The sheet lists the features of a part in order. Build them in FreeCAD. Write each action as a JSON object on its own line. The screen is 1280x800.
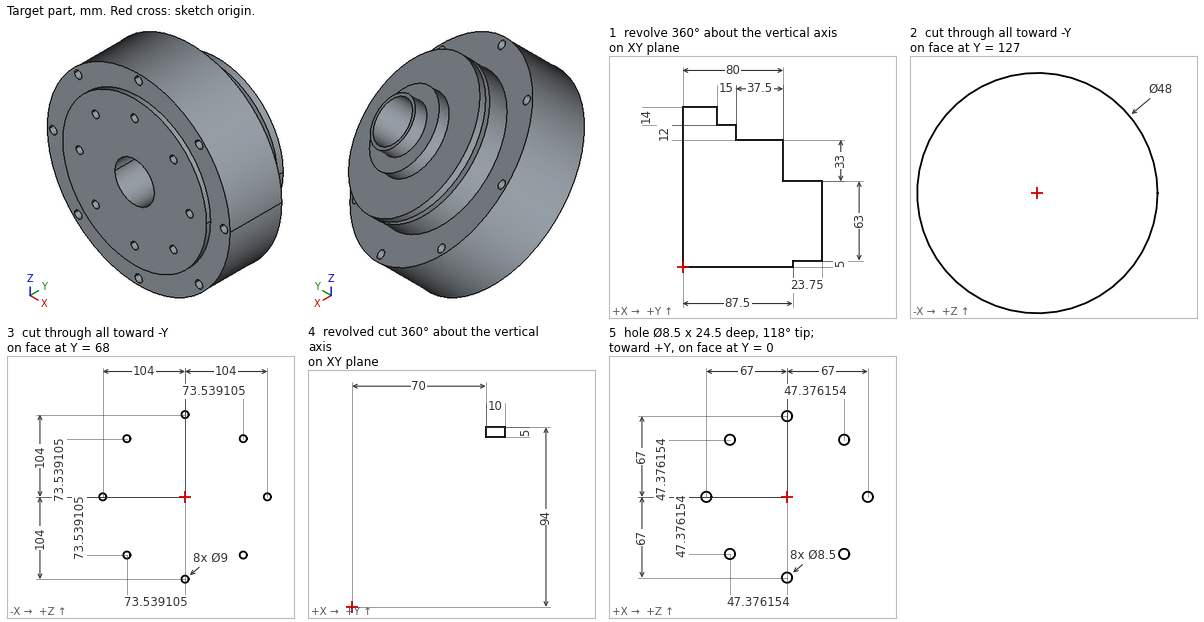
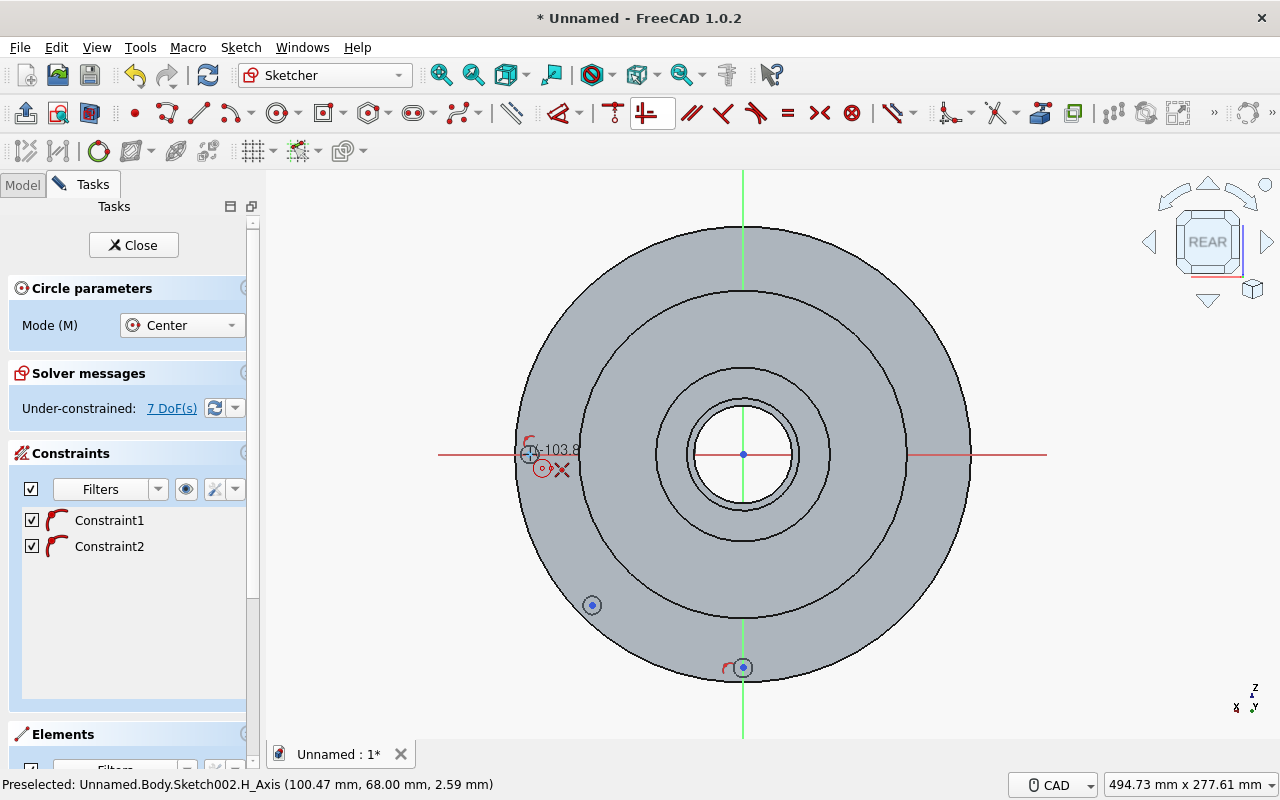
{"action": "scroll", "coordinate": [581, 331], "scroll_direction": "up", "scroll_amount": 6}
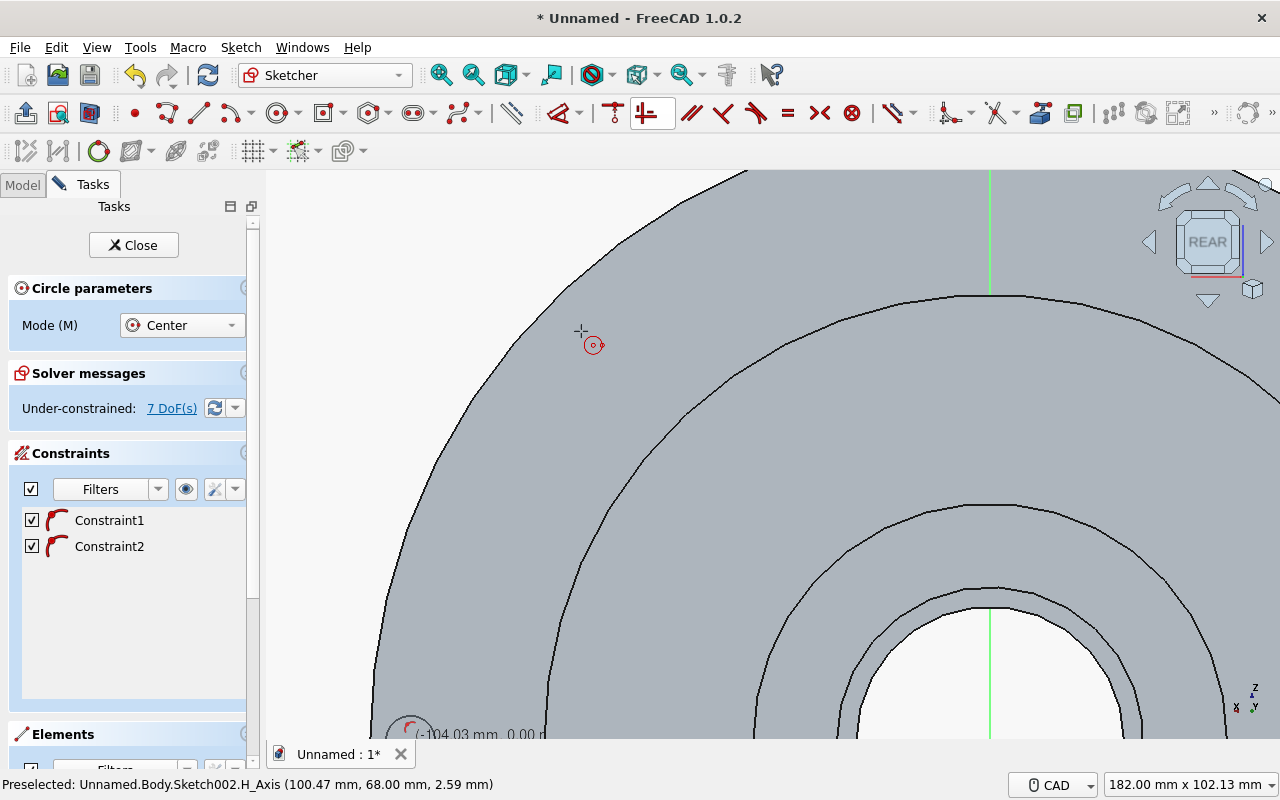
{"action": "left_click", "coordinate": [580, 331]}
{"action": "left_click", "coordinate": [598, 313]}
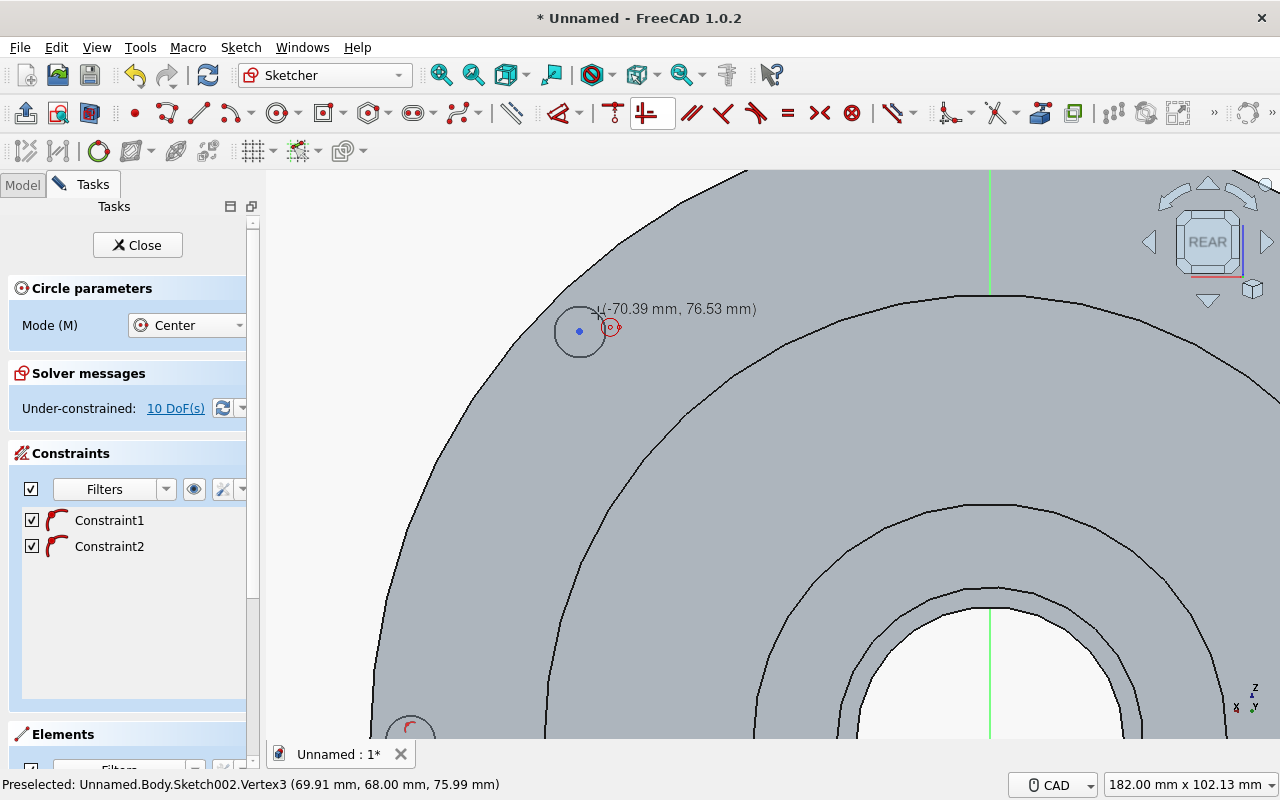
{"action": "scroll", "coordinate": [581, 331], "scroll_direction": "down", "scroll_amount": 6}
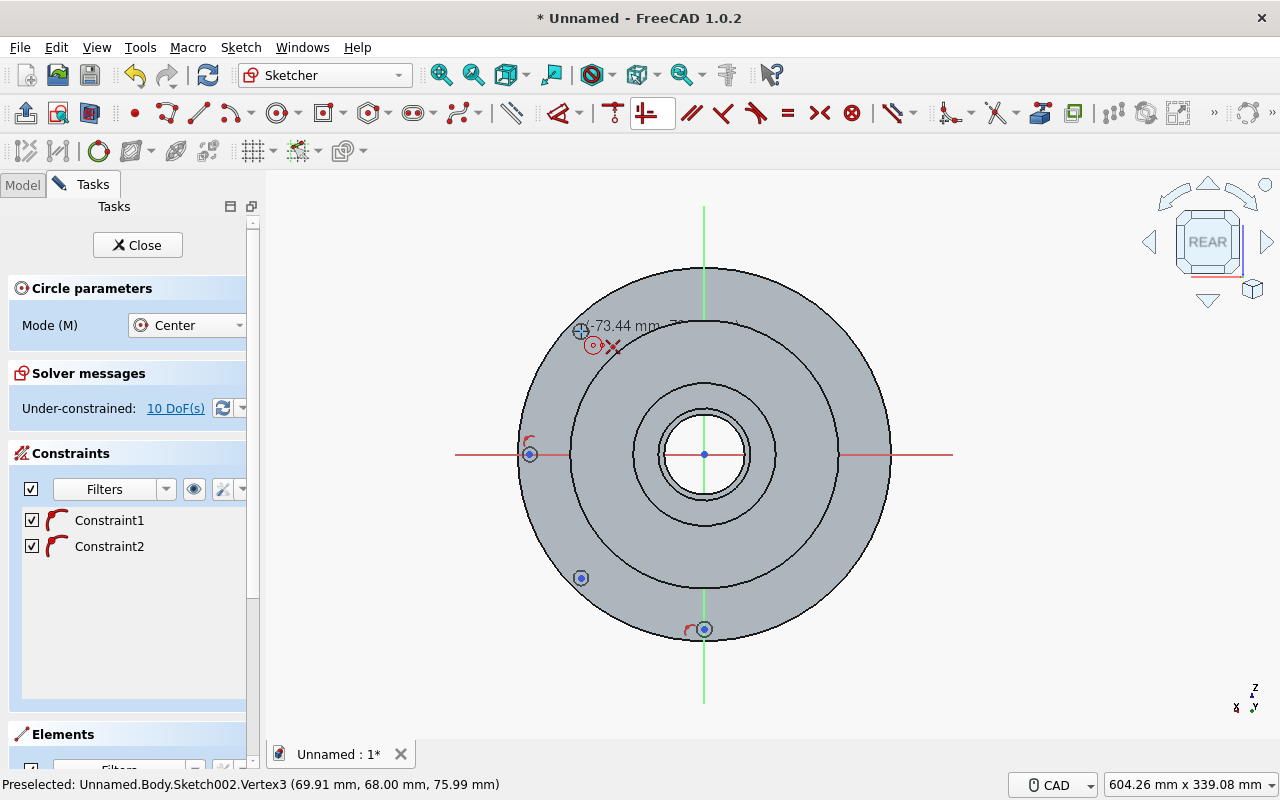
{"action": "scroll", "coordinate": [704, 280], "scroll_direction": "up", "scroll_amount": 6}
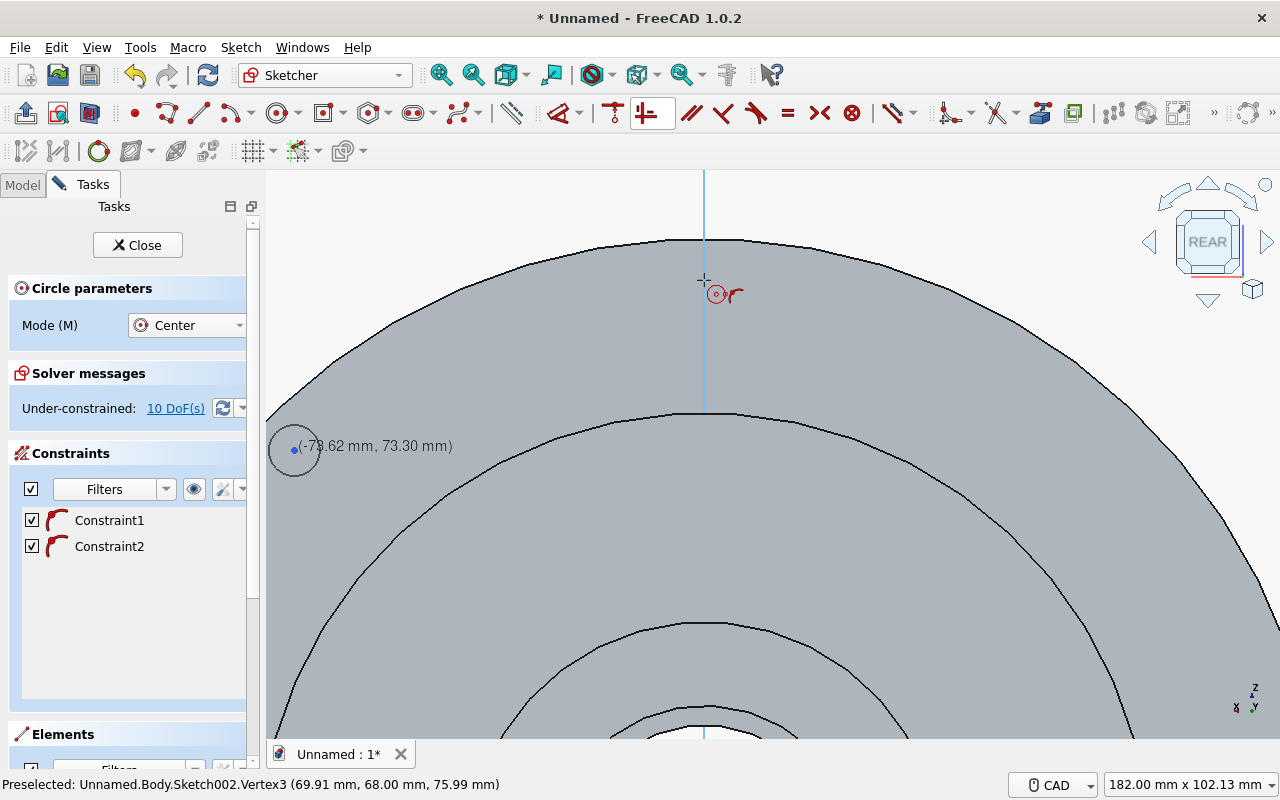
{"action": "left_click", "coordinate": [704, 279]}
{"action": "left_click", "coordinate": [722, 262]}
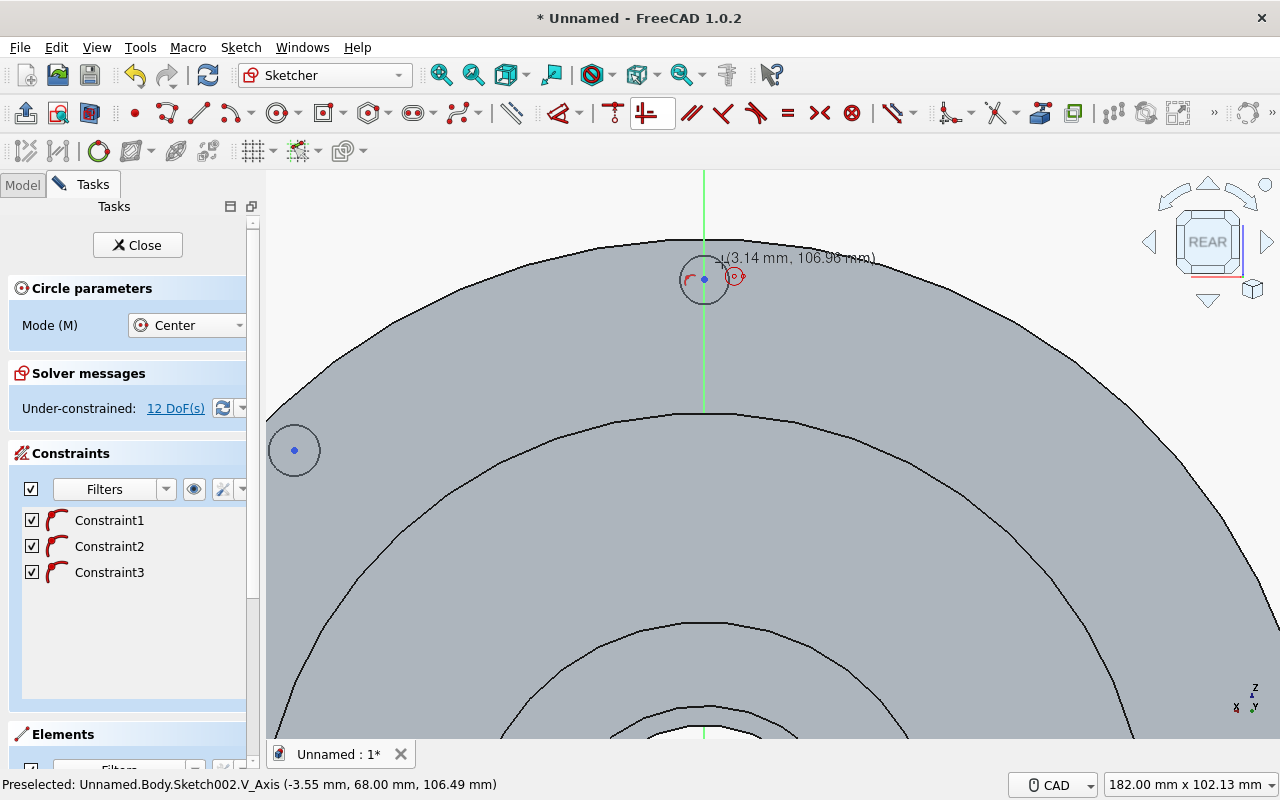
{"action": "left_click", "coordinate": [1114, 449]}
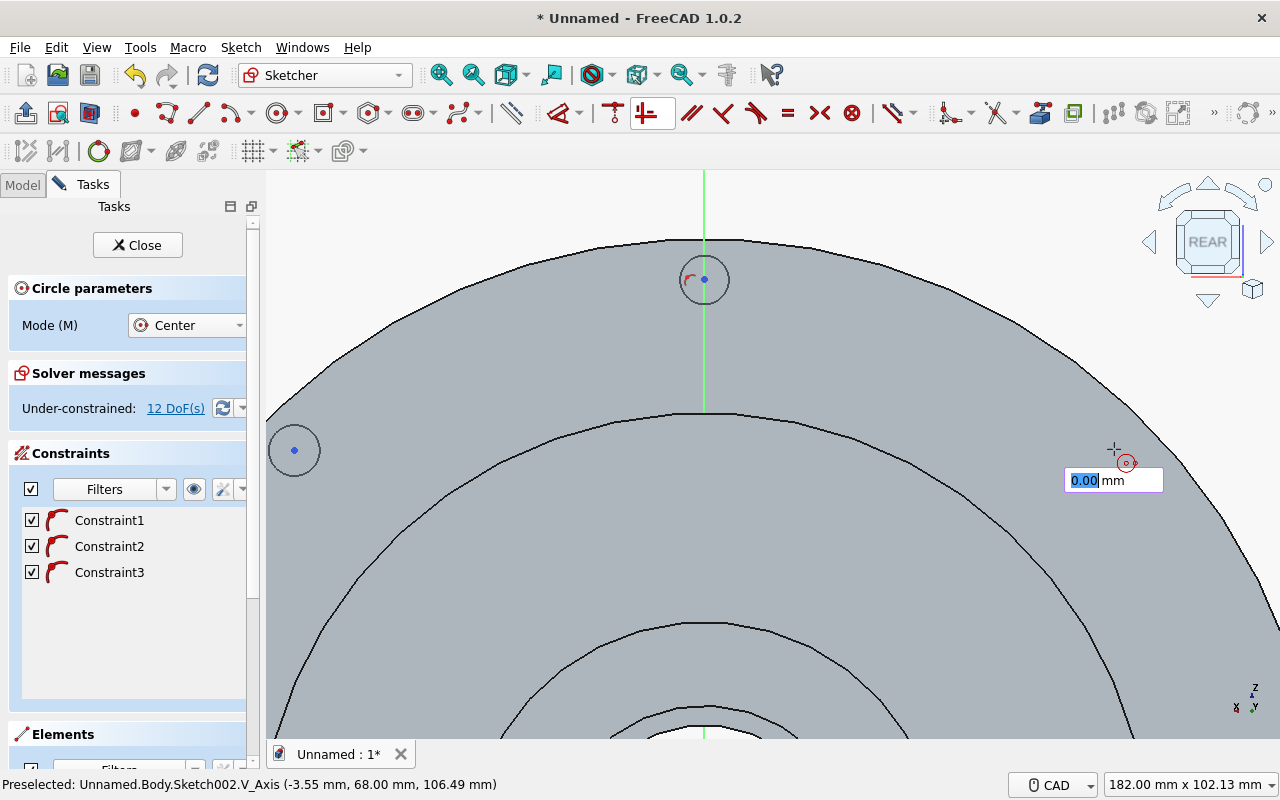
{"action": "scroll", "coordinate": [705, 280], "scroll_direction": "down", "scroll_amount": 6}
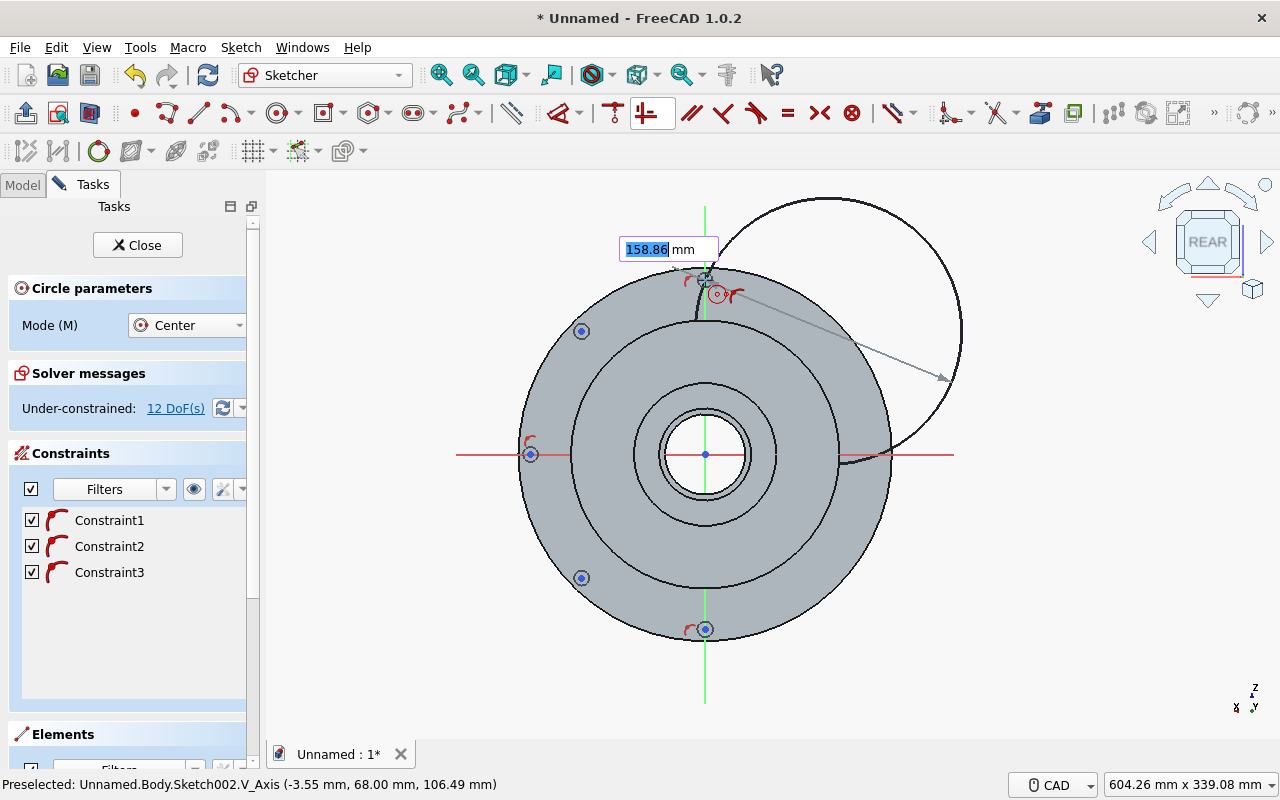
{"action": "scroll", "coordinate": [834, 326], "scroll_direction": "up", "scroll_amount": 4}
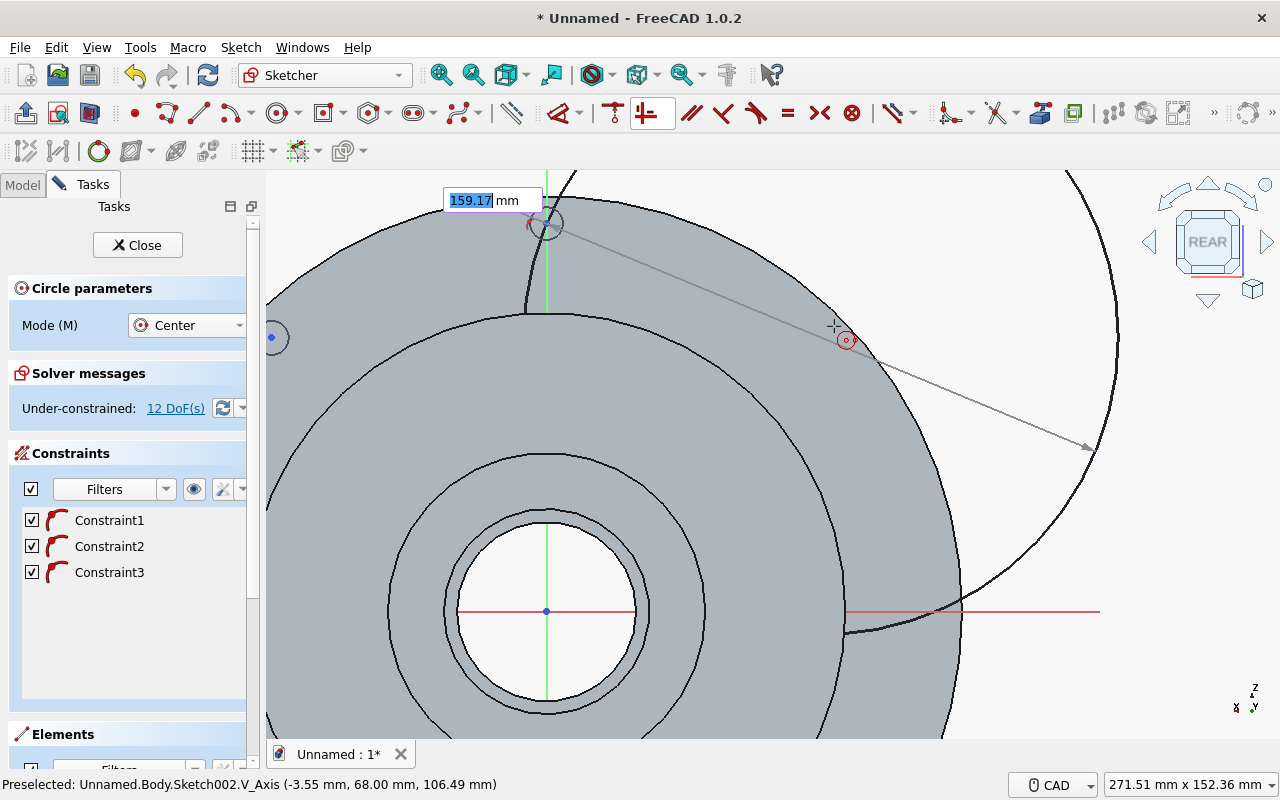
{"action": "left_click", "coordinate": [833, 325]}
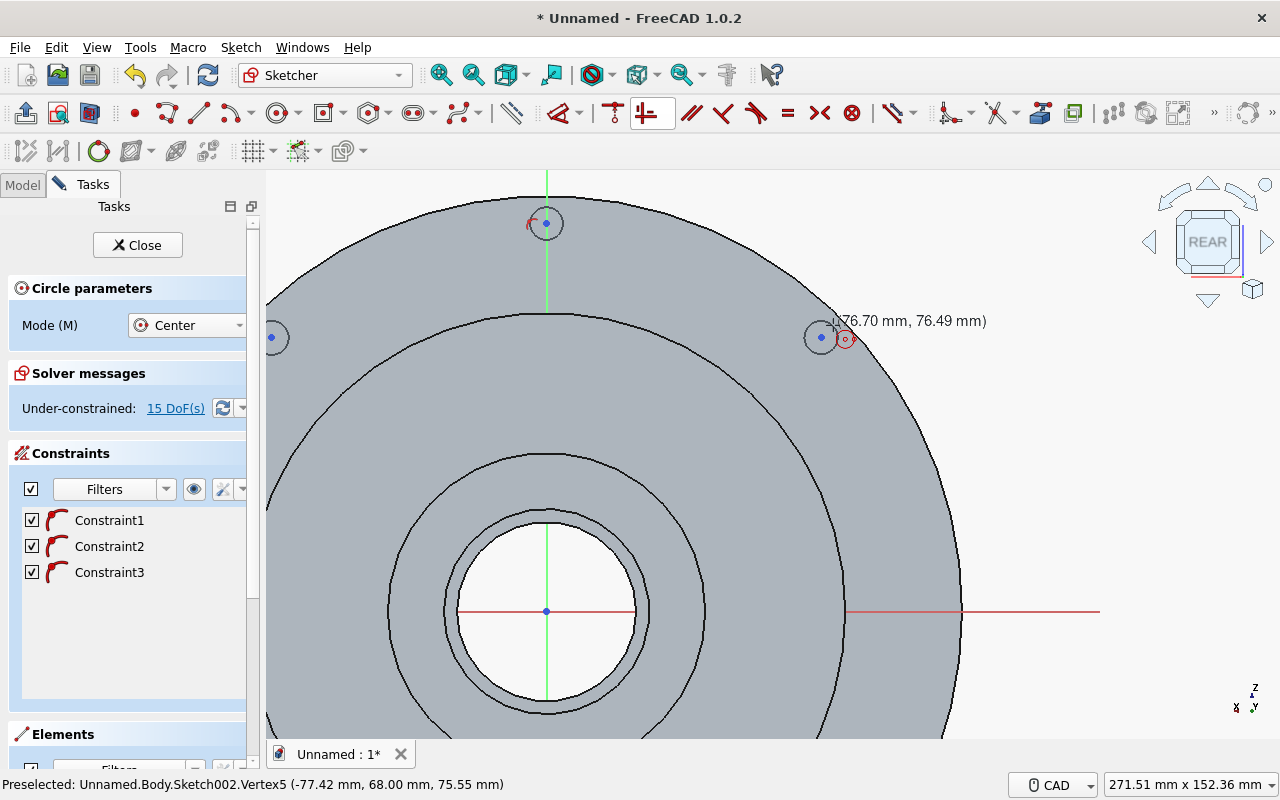
{"action": "scroll", "coordinate": [935, 612], "scroll_direction": "up", "scroll_amount": 2}